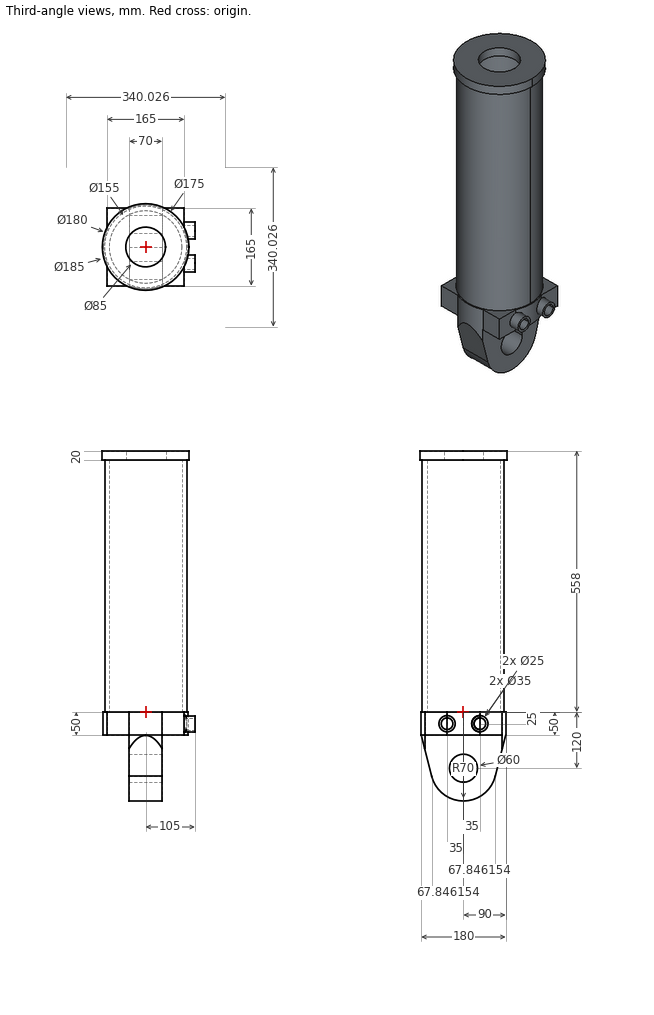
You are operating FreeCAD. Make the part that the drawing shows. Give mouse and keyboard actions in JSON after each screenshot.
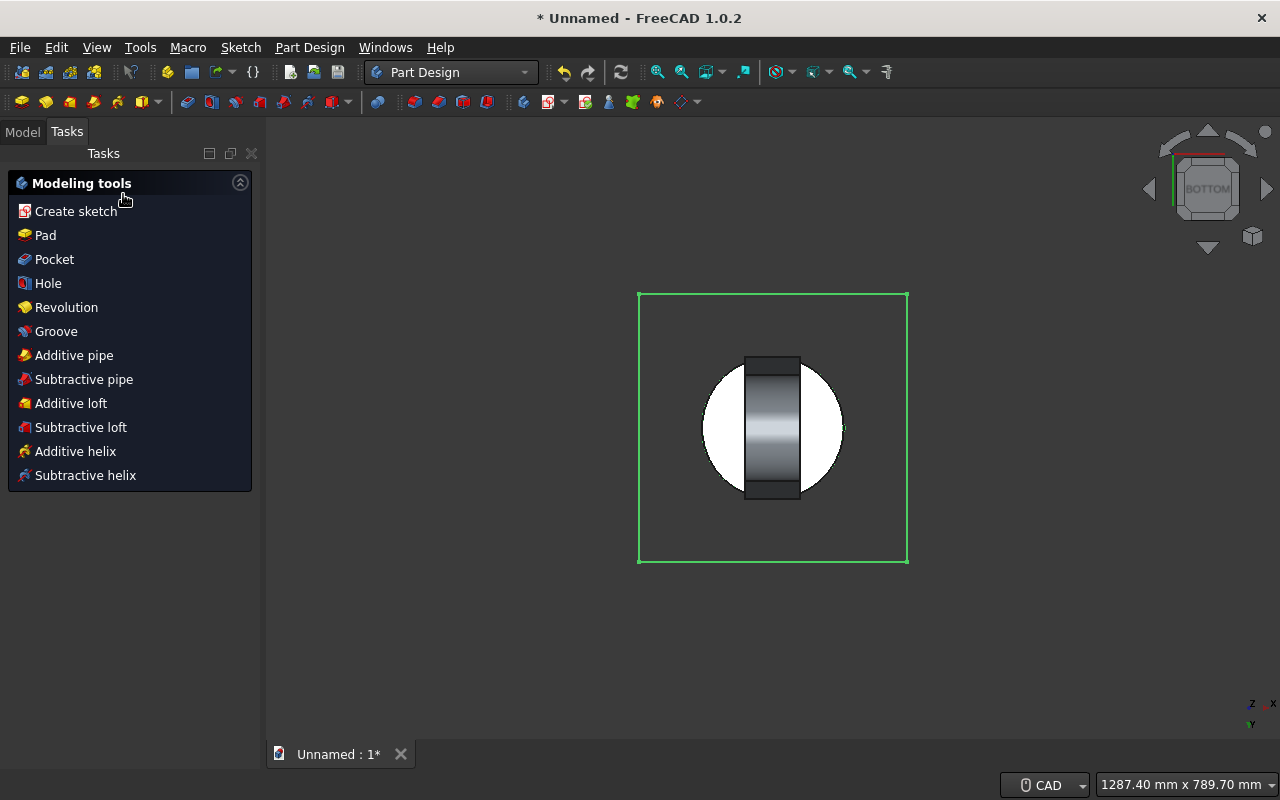
{"action": "left_click", "coordinate": [188, 102]}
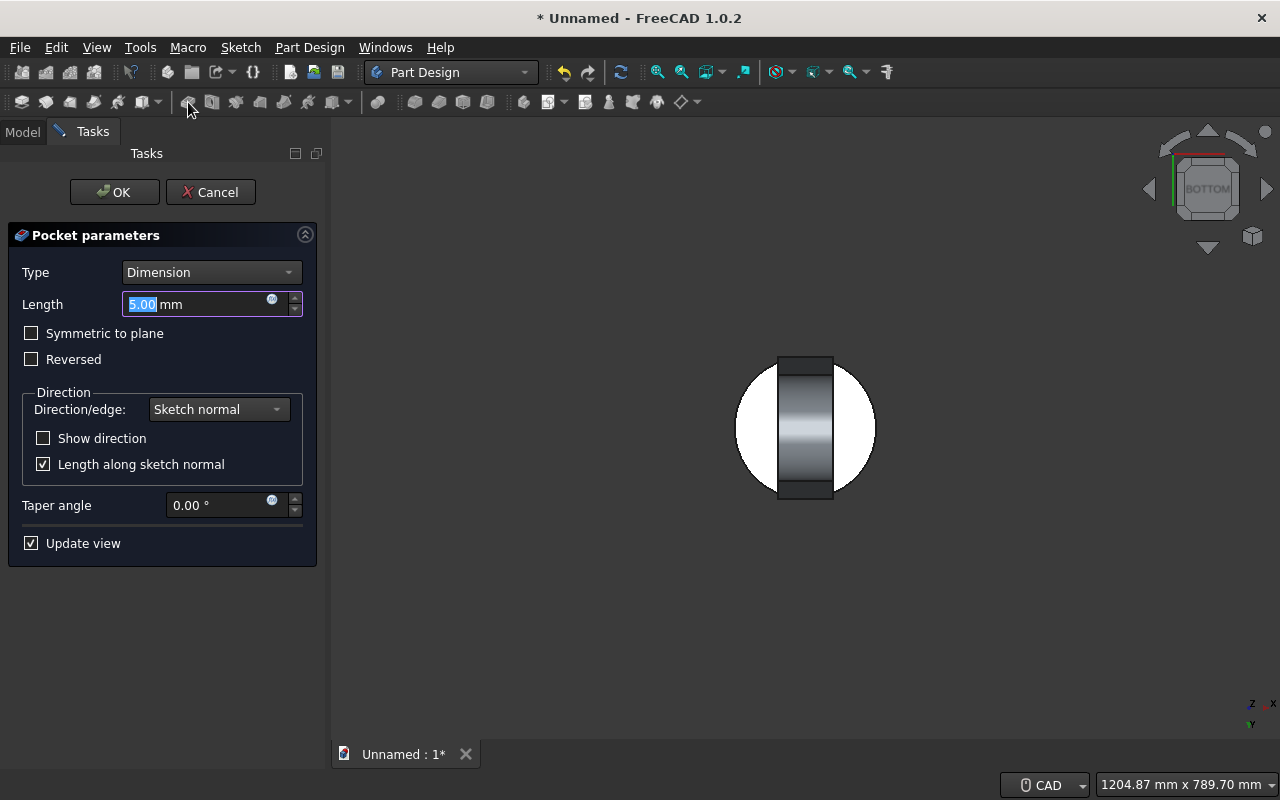
{"action": "left_click", "coordinate": [212, 272]}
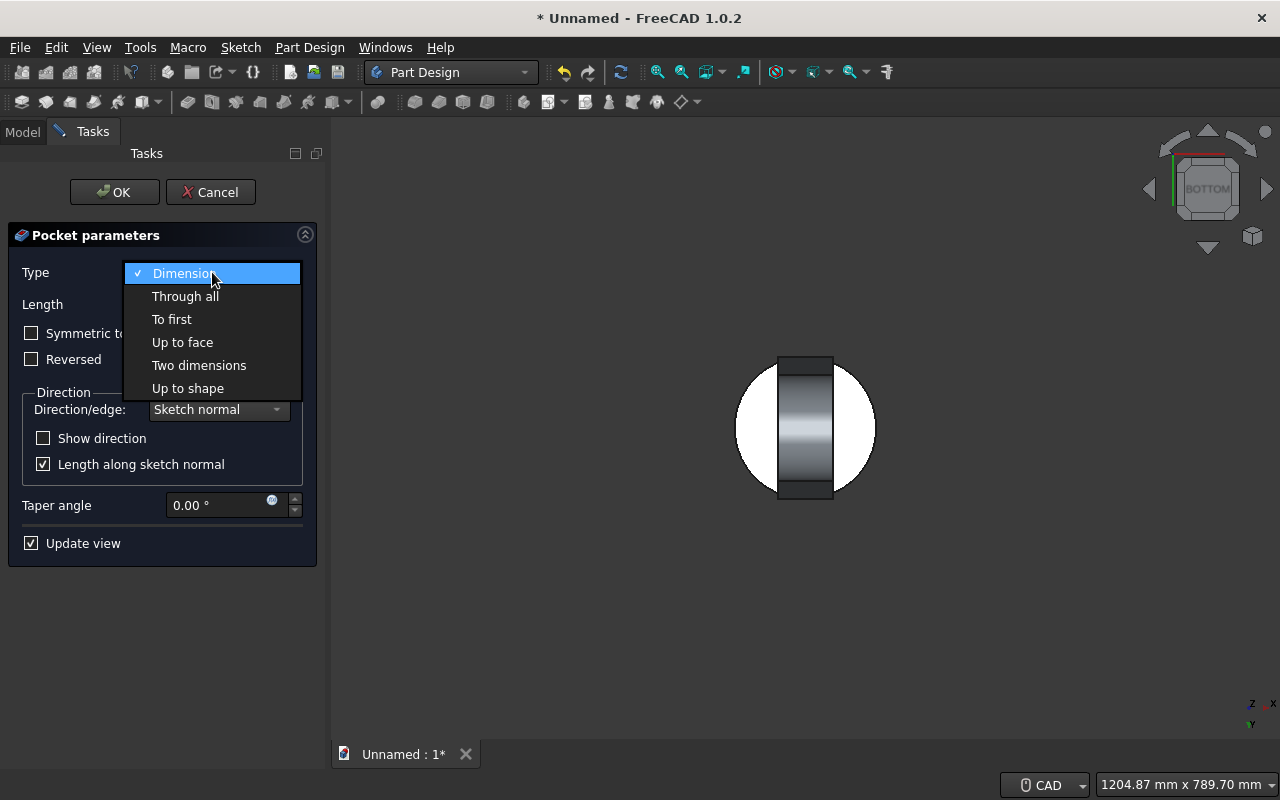
{"action": "left_click", "coordinate": [212, 296]}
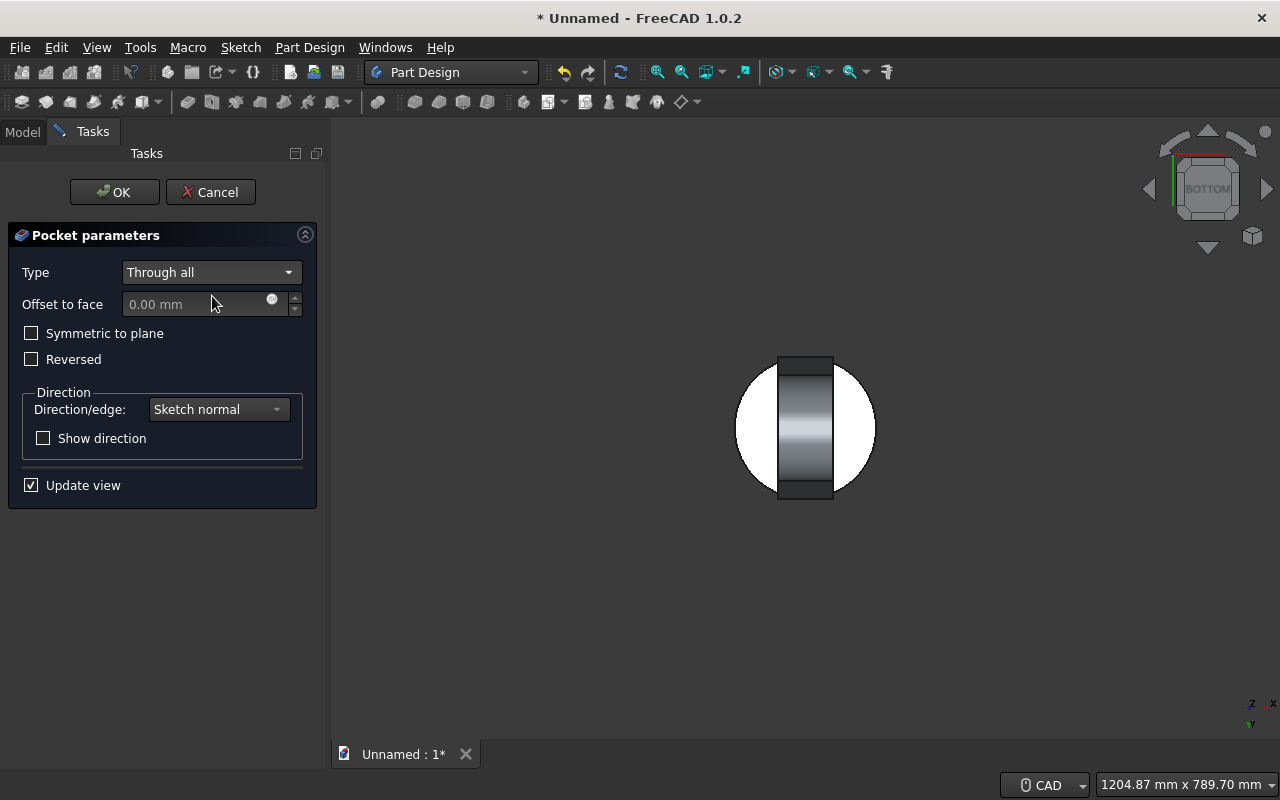
{"action": "left_click", "coordinate": [30, 359]}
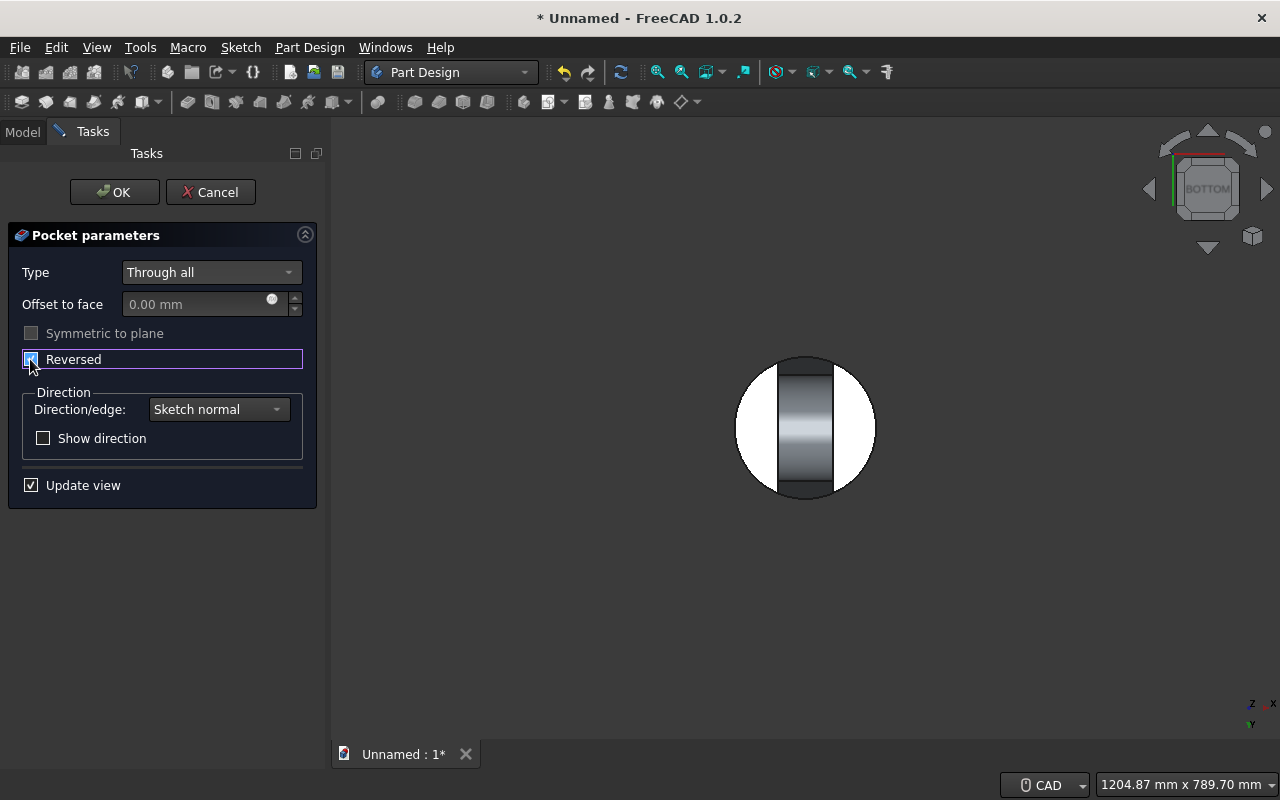
{"action": "left_click", "coordinate": [115, 192]}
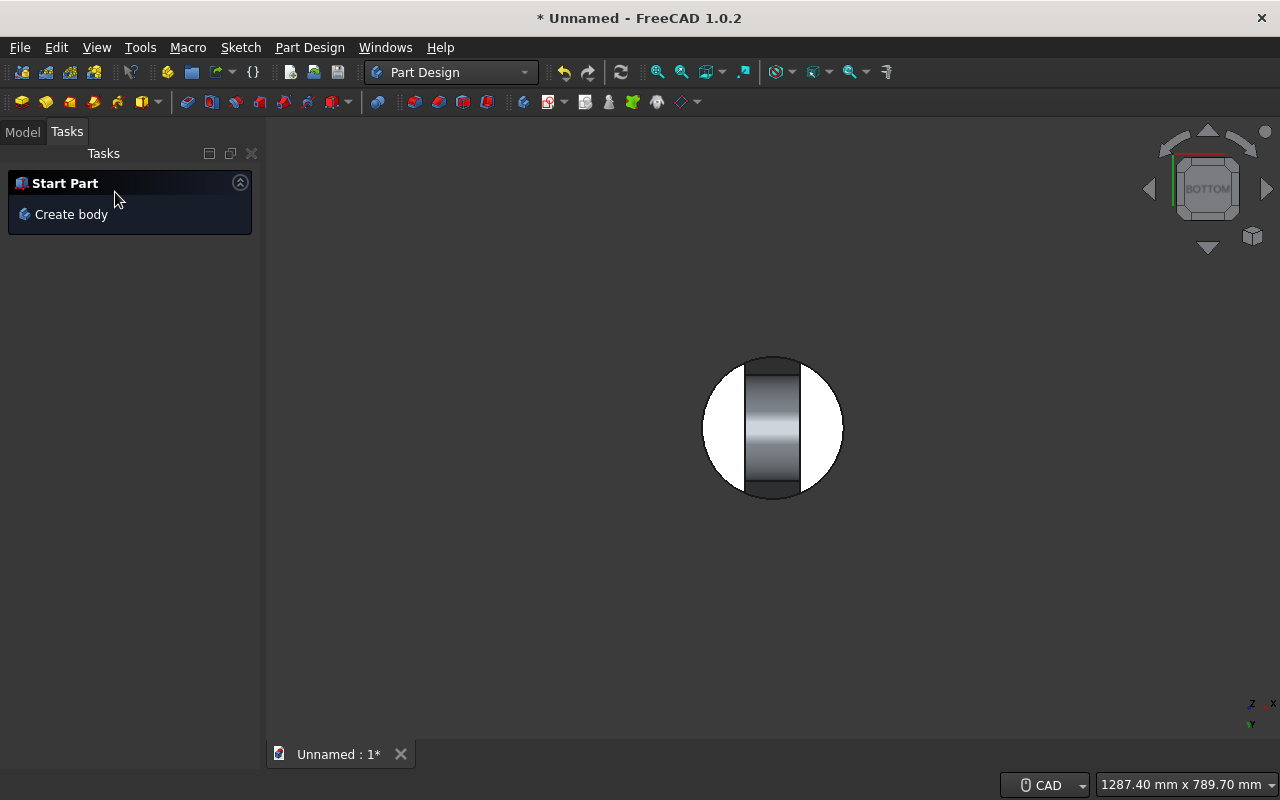
{"action": "key", "text": "v f"}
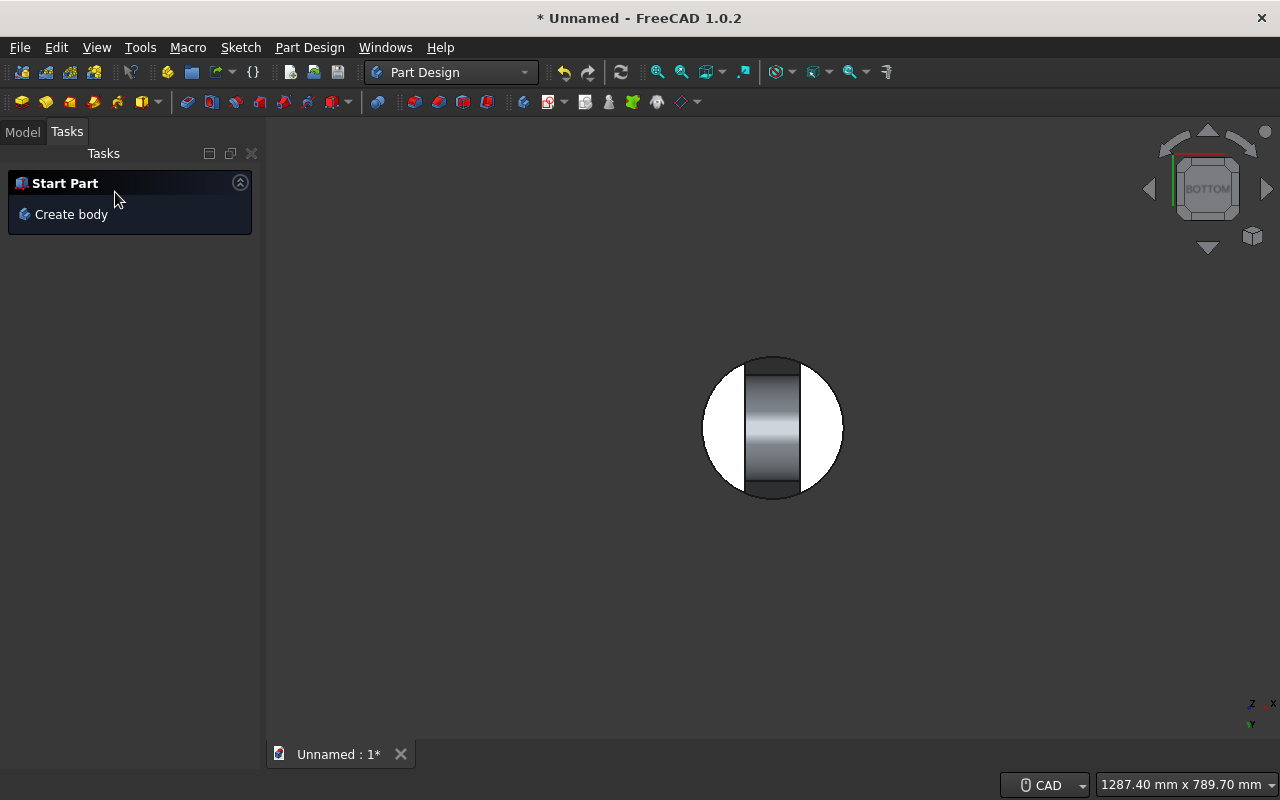
{"action": "left_click", "coordinate": [548, 102]}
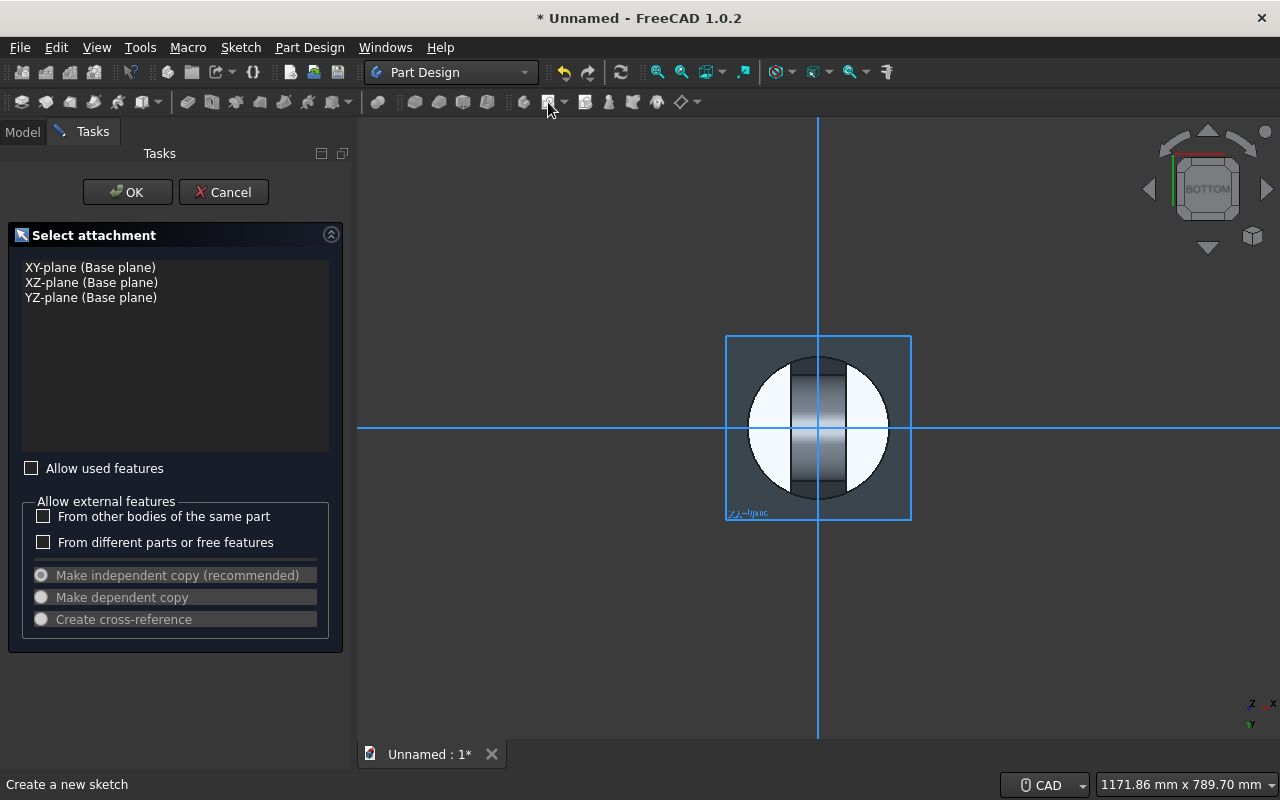
{"action": "left_click", "coordinate": [82, 298]}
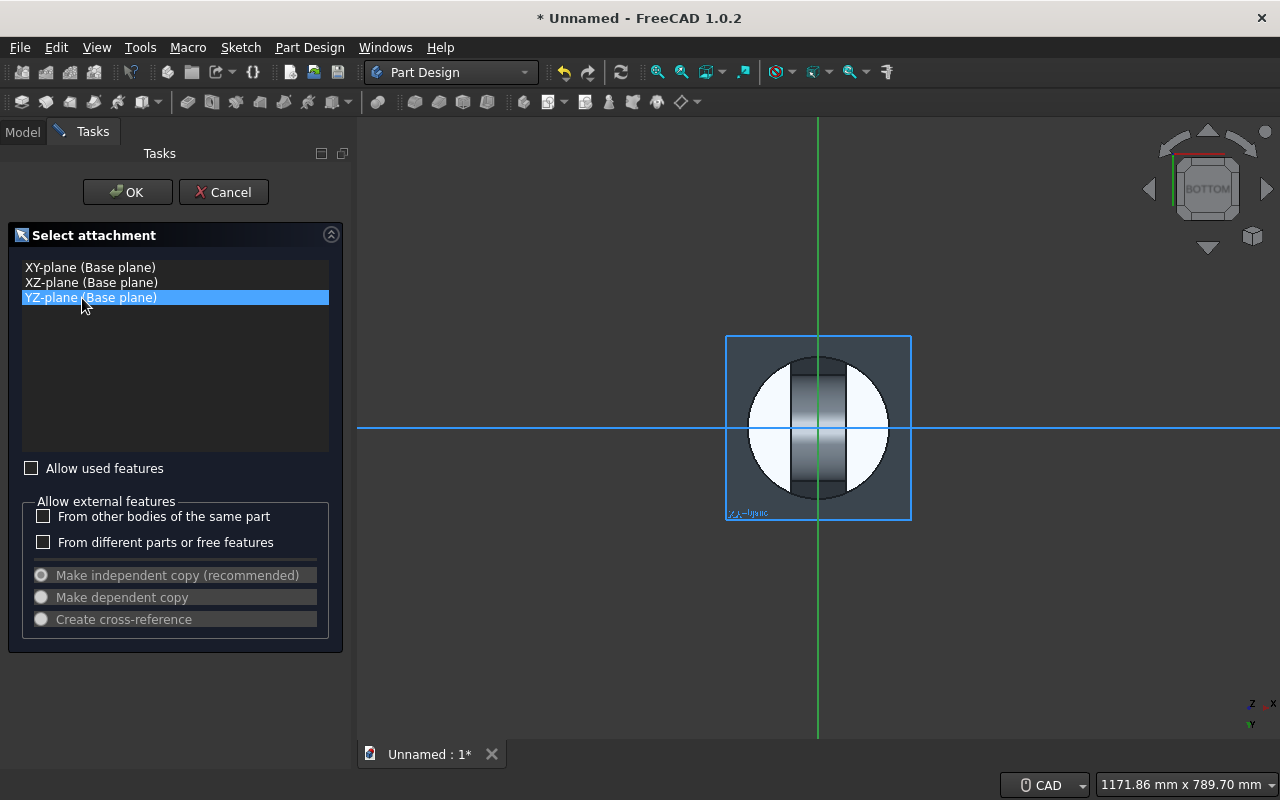
{"action": "left_click", "coordinate": [128, 192]}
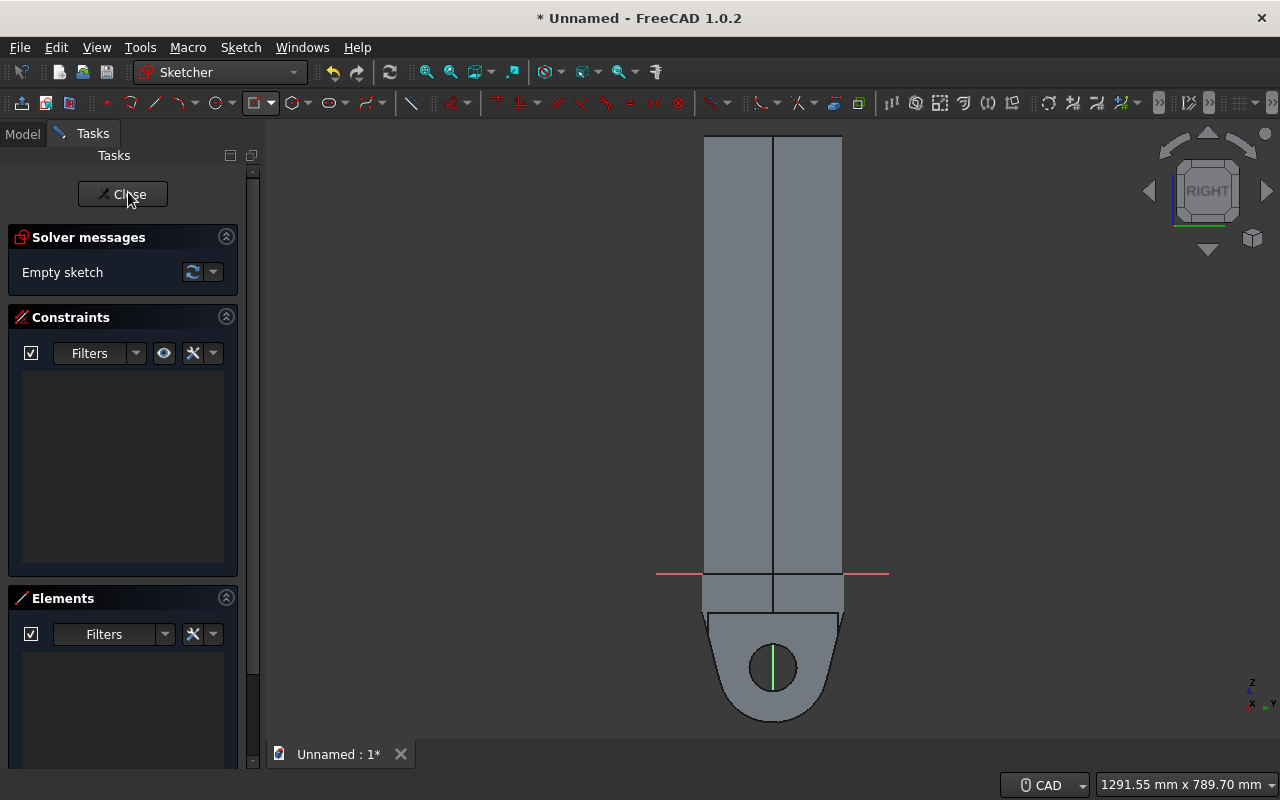
{"action": "left_click", "coordinate": [70, 104]}